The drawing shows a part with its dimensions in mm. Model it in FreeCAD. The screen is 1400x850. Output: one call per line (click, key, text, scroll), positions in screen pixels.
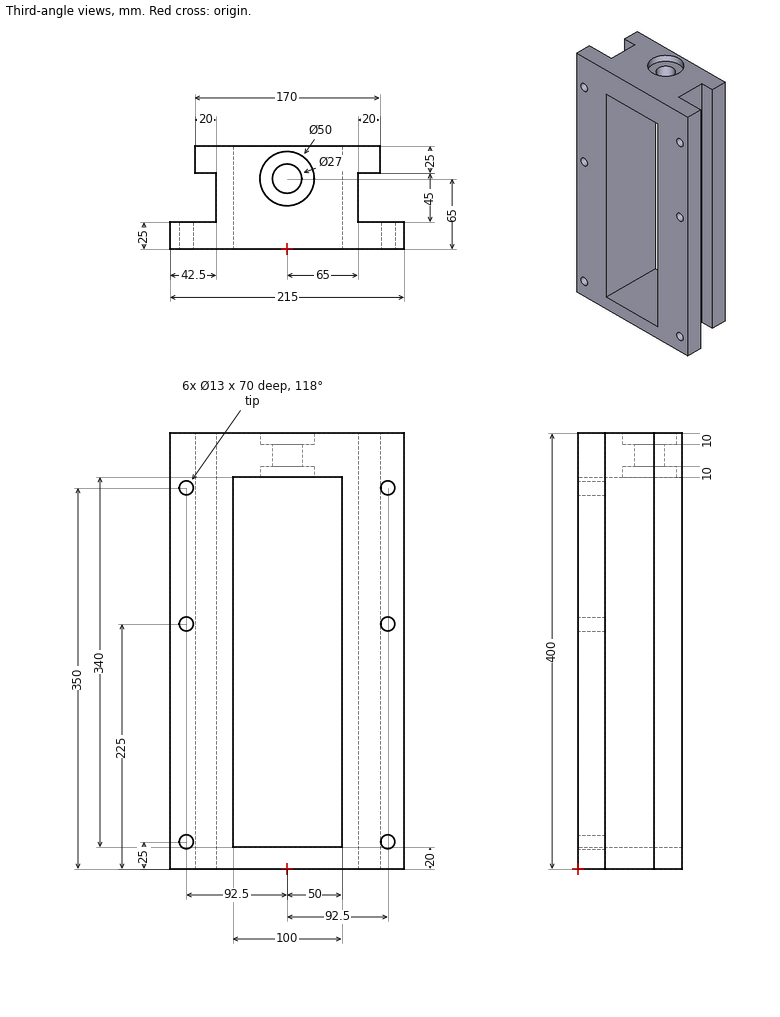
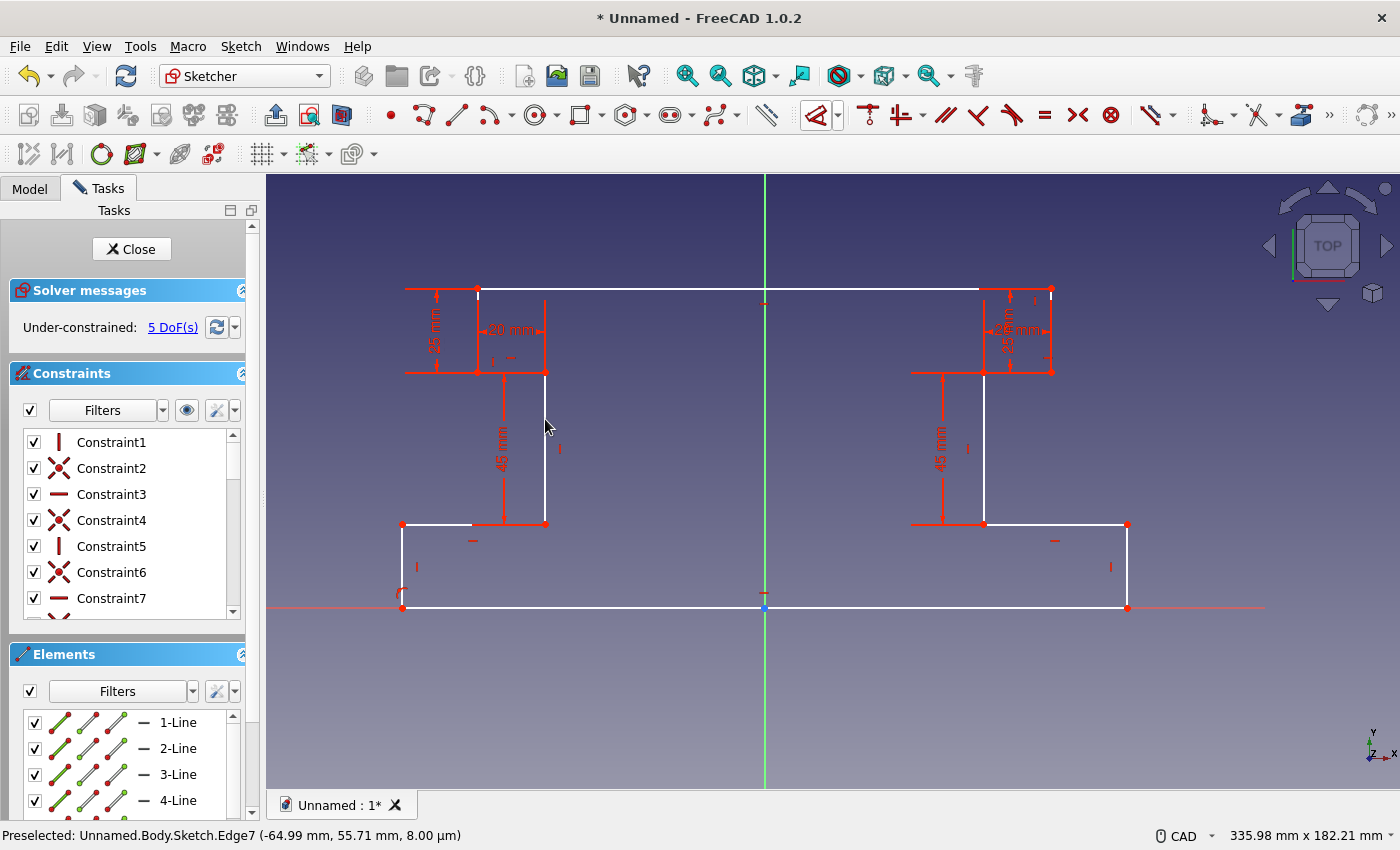
click(402, 550)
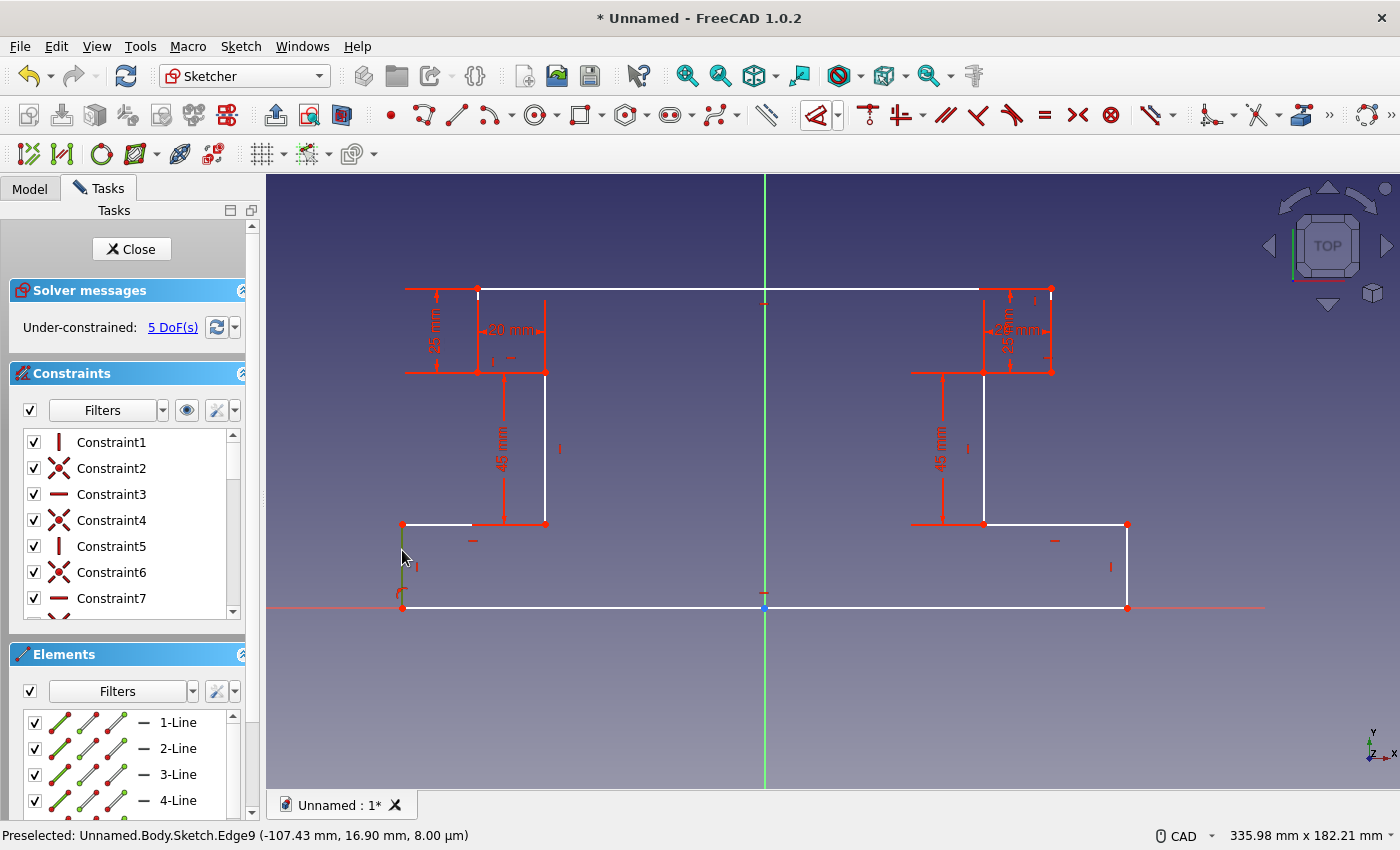
key(i)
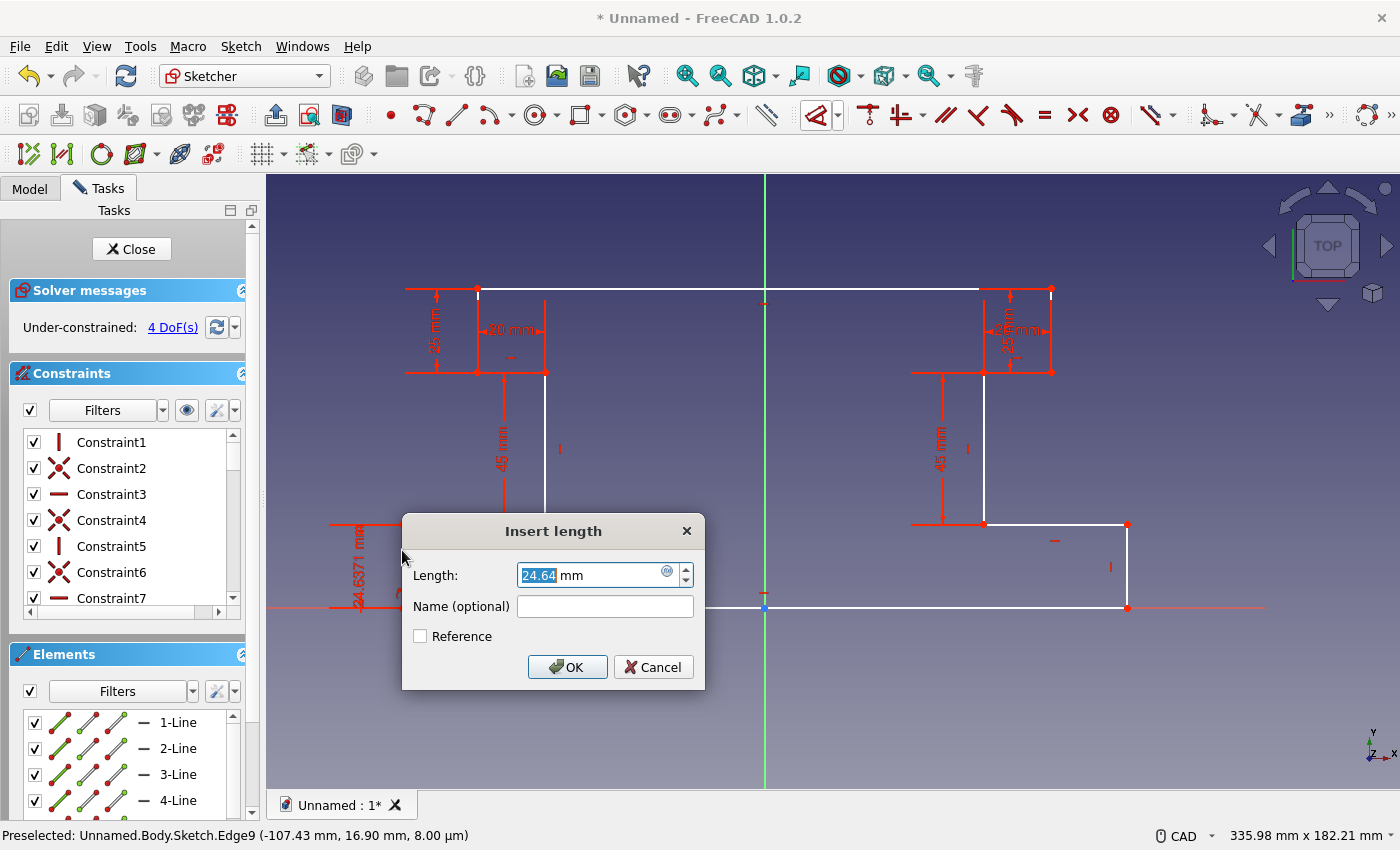
text(25)
key(Return)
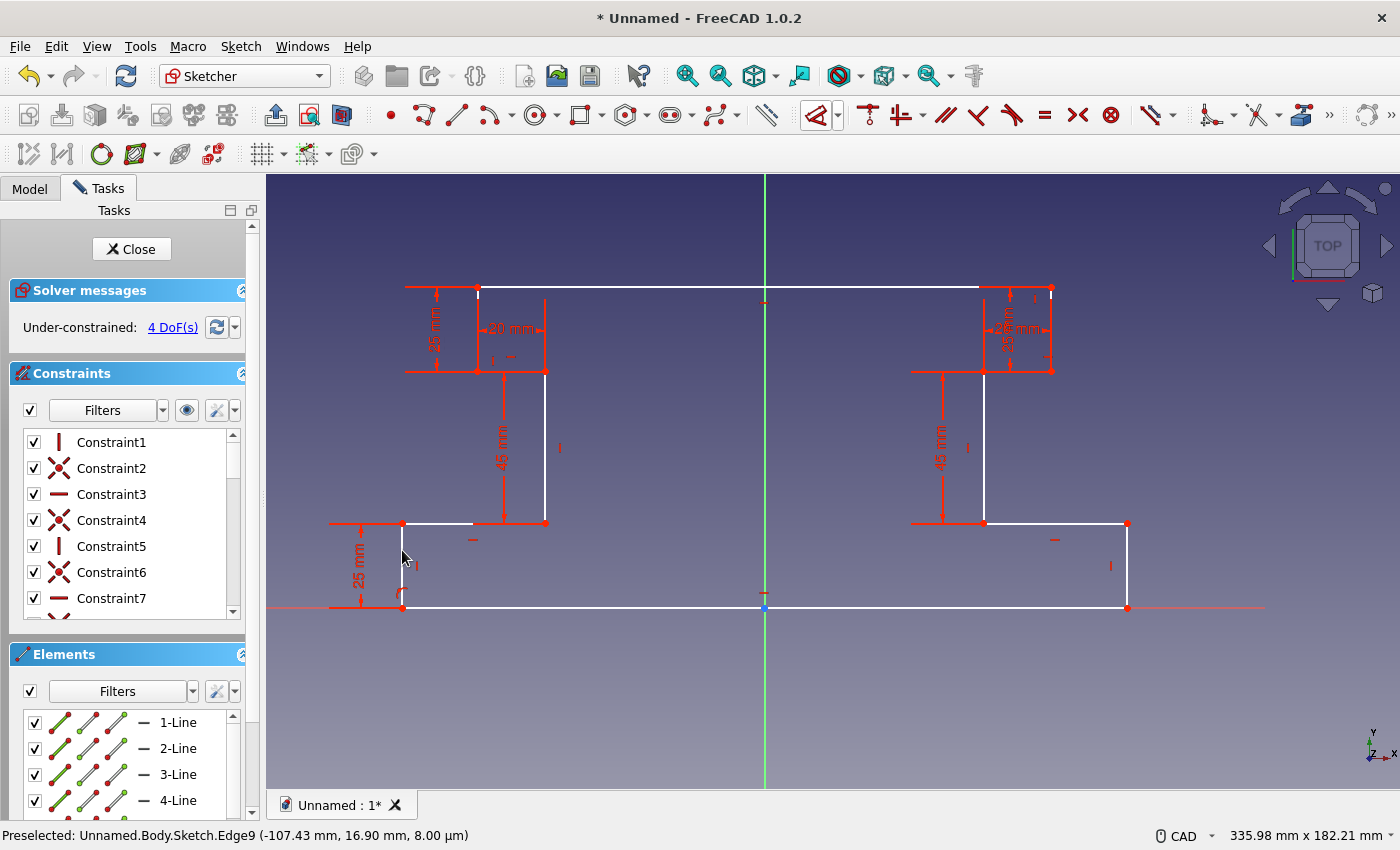
click(879, 287)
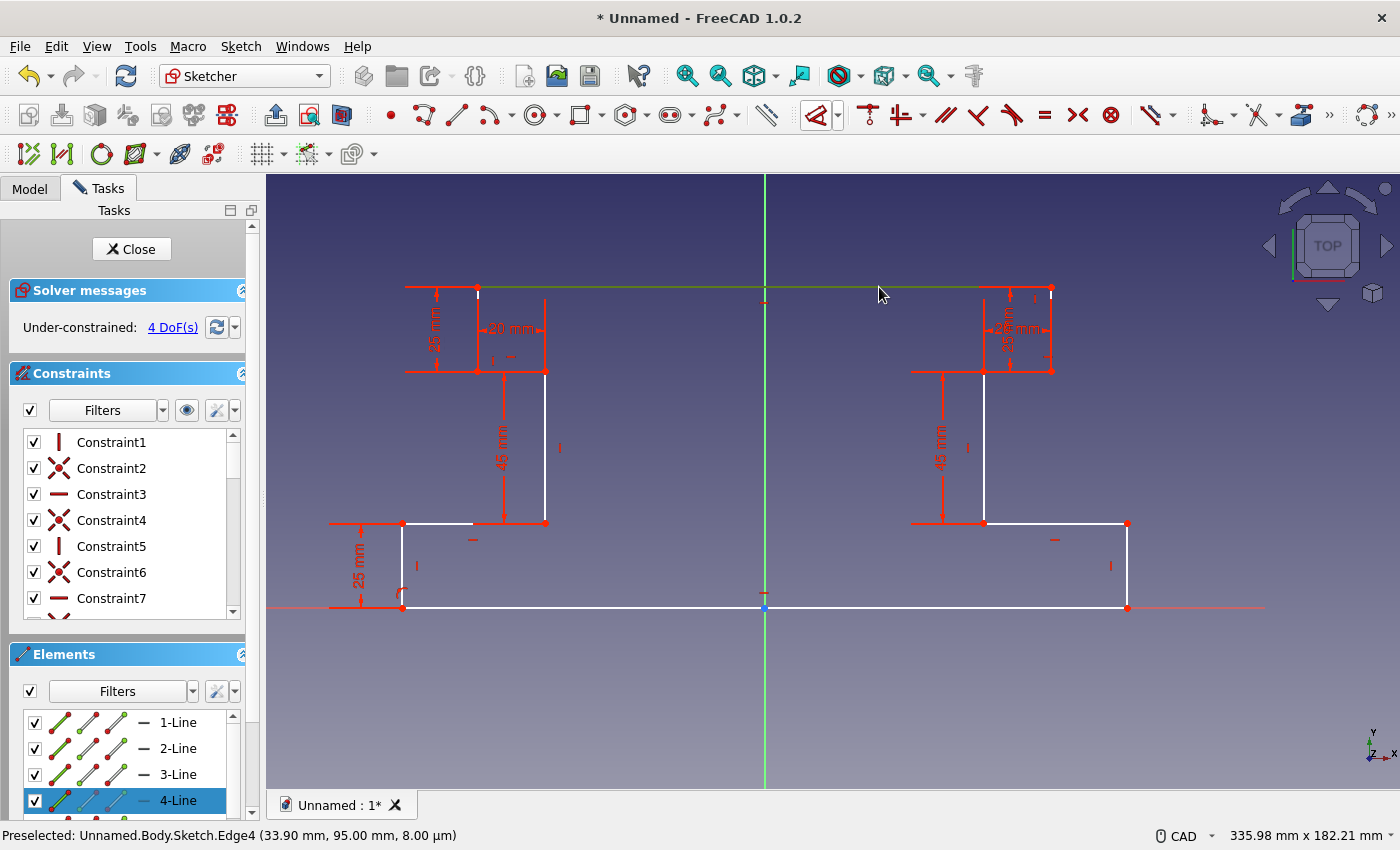
key(l)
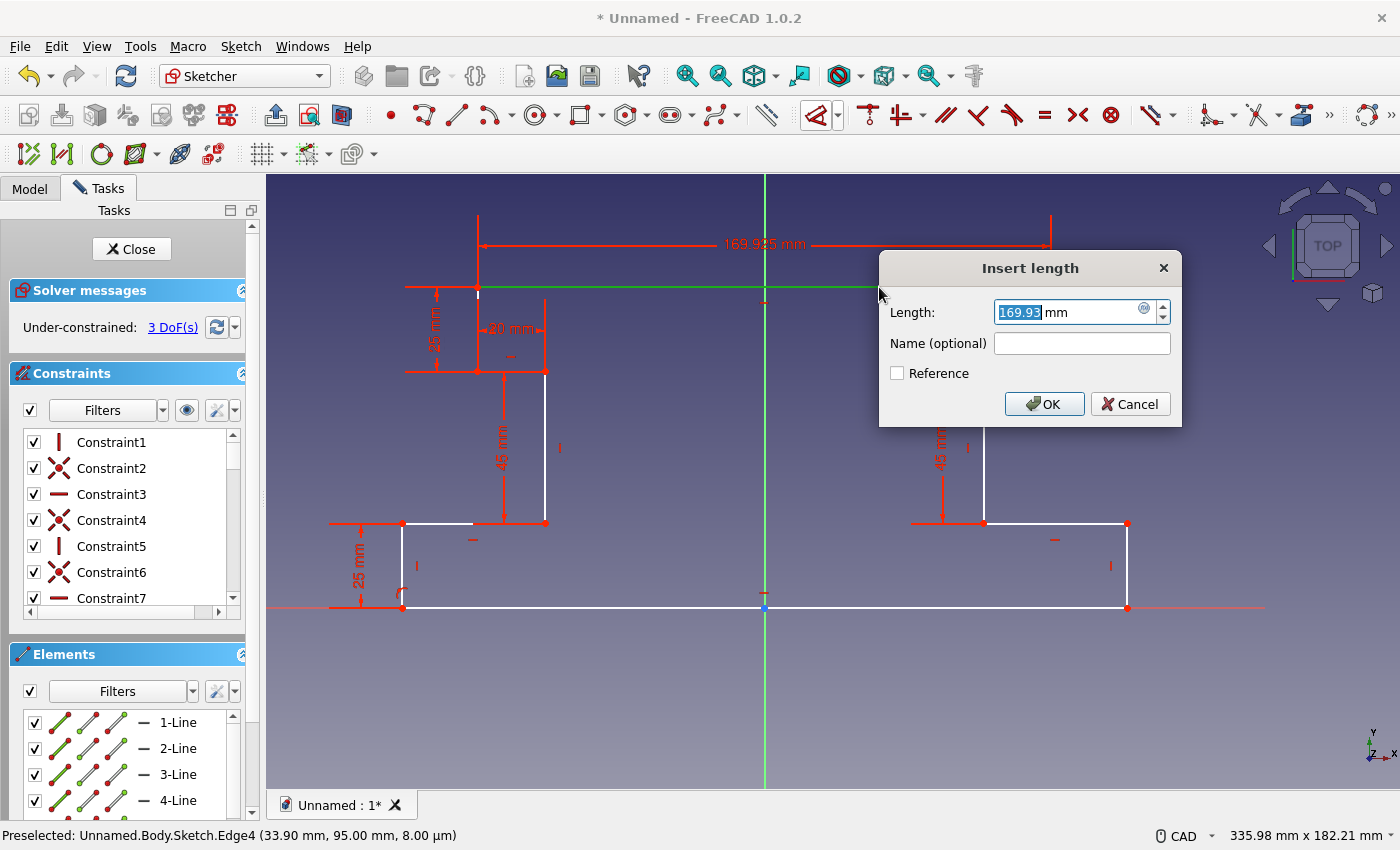
text(170)
key(Return)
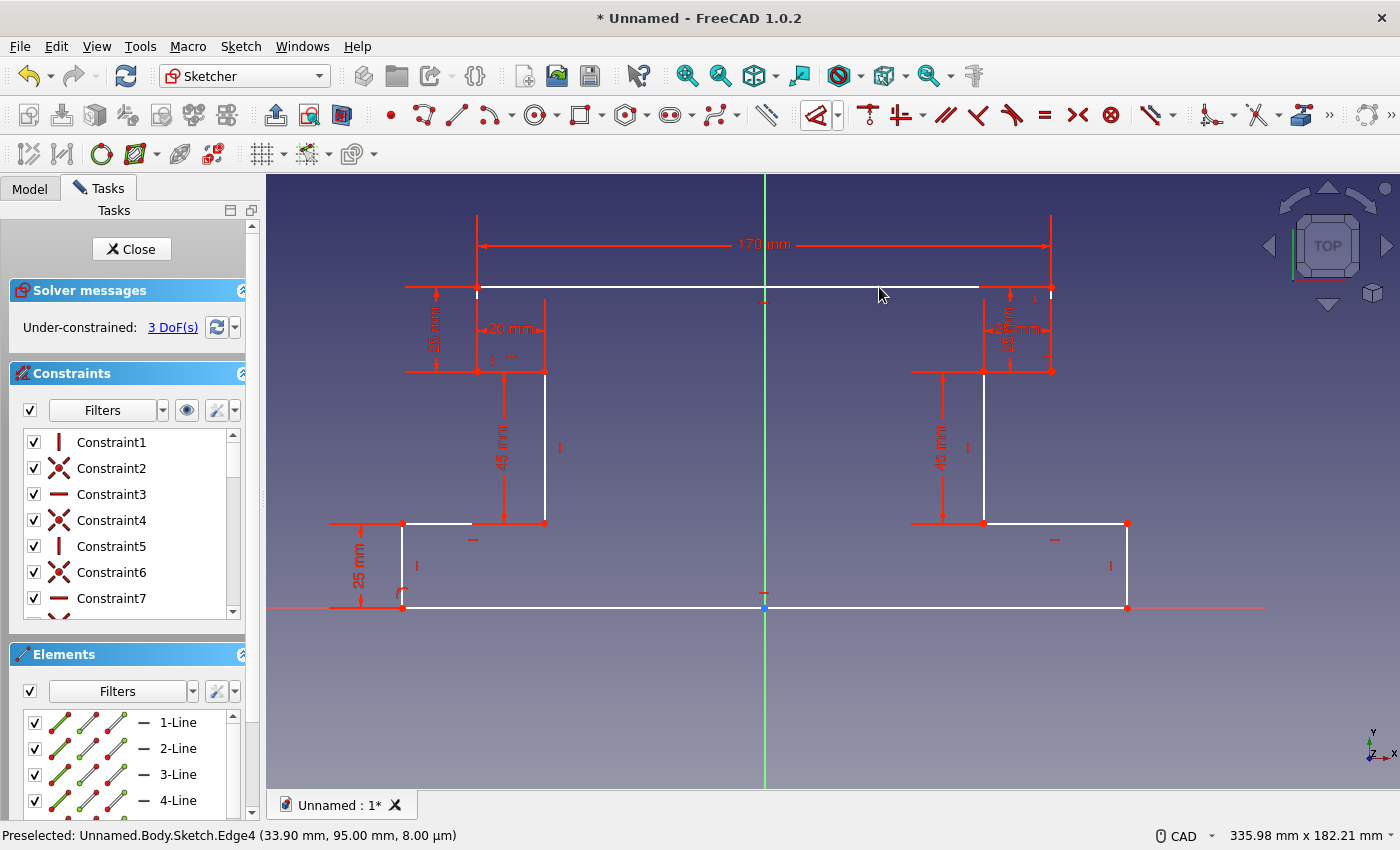
click(620, 608)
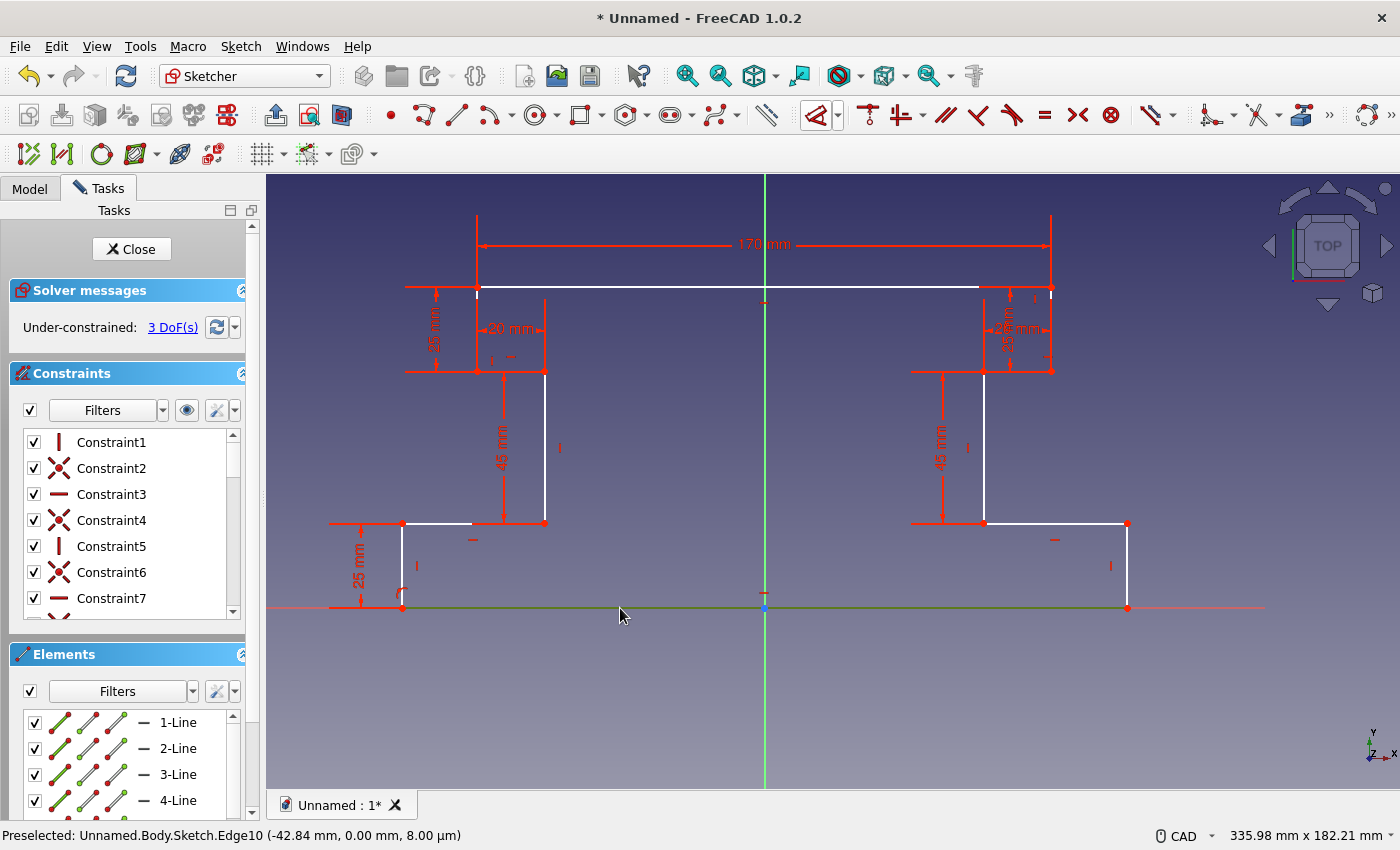
key(l)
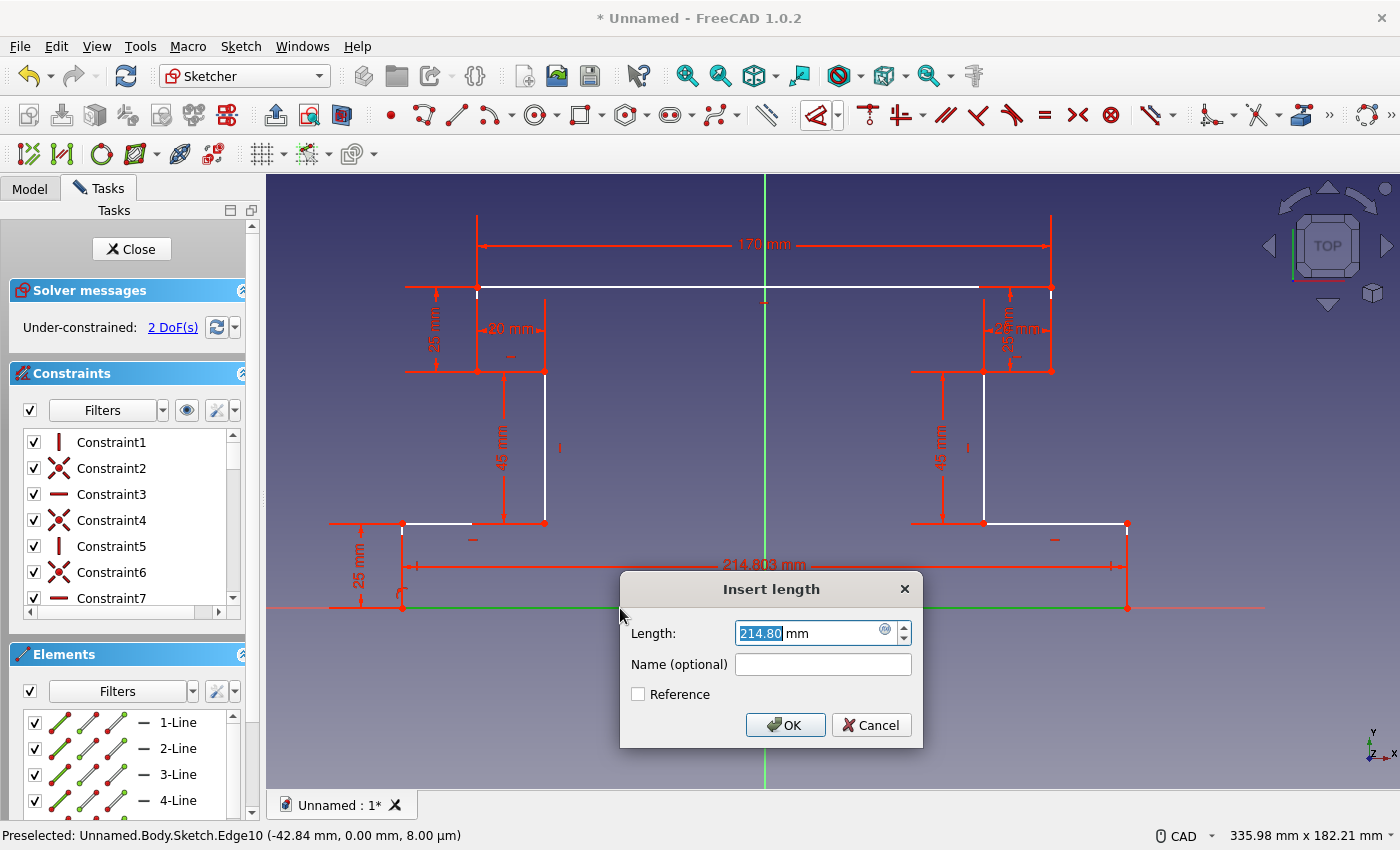
text(215)
key(Return)